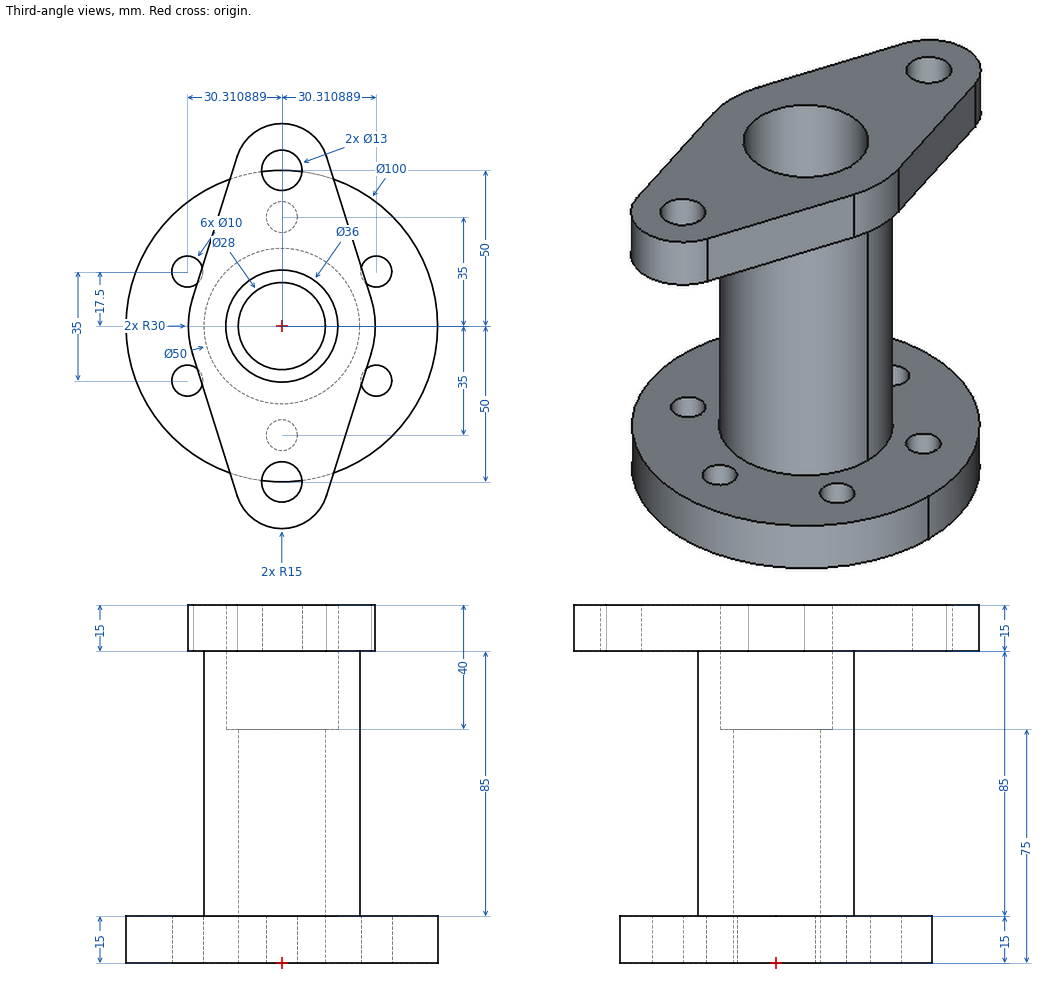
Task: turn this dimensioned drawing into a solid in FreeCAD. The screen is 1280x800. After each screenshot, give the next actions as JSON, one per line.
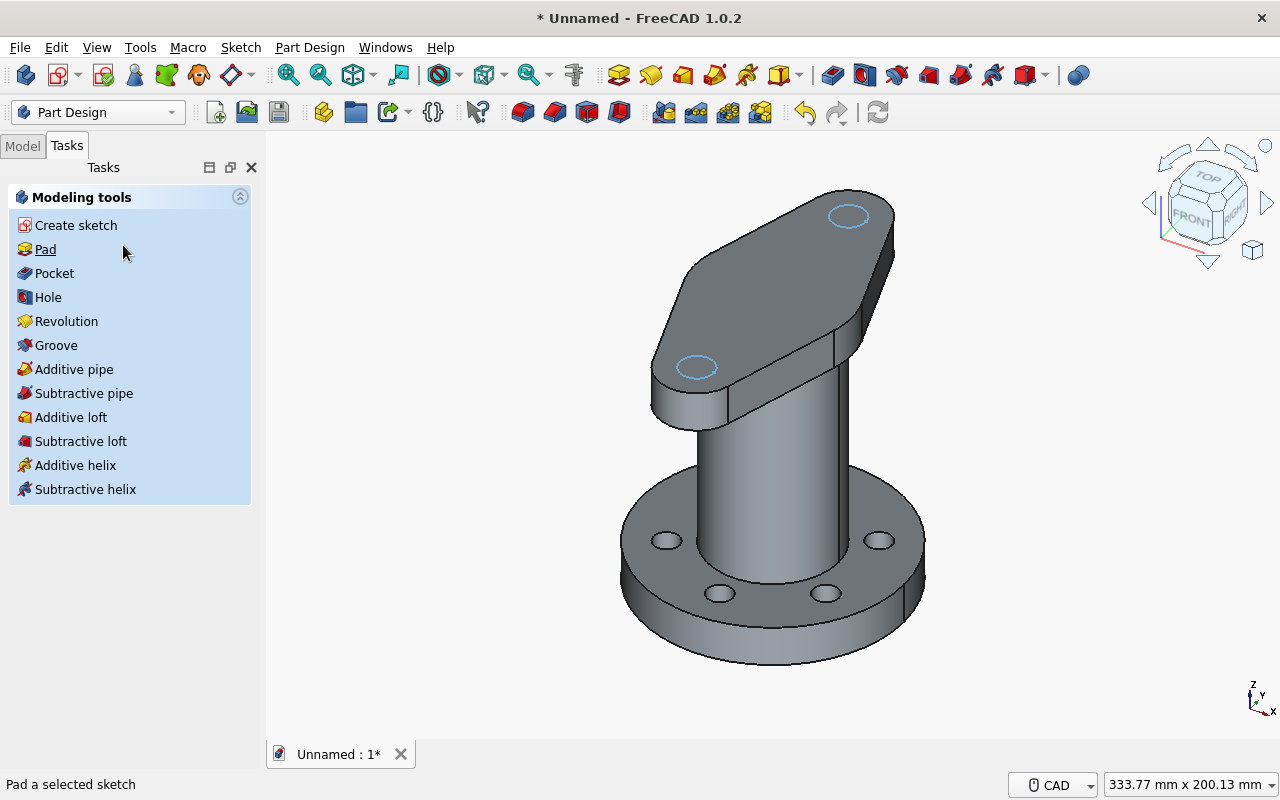
{"action": "left_click", "coordinate": [834, 76]}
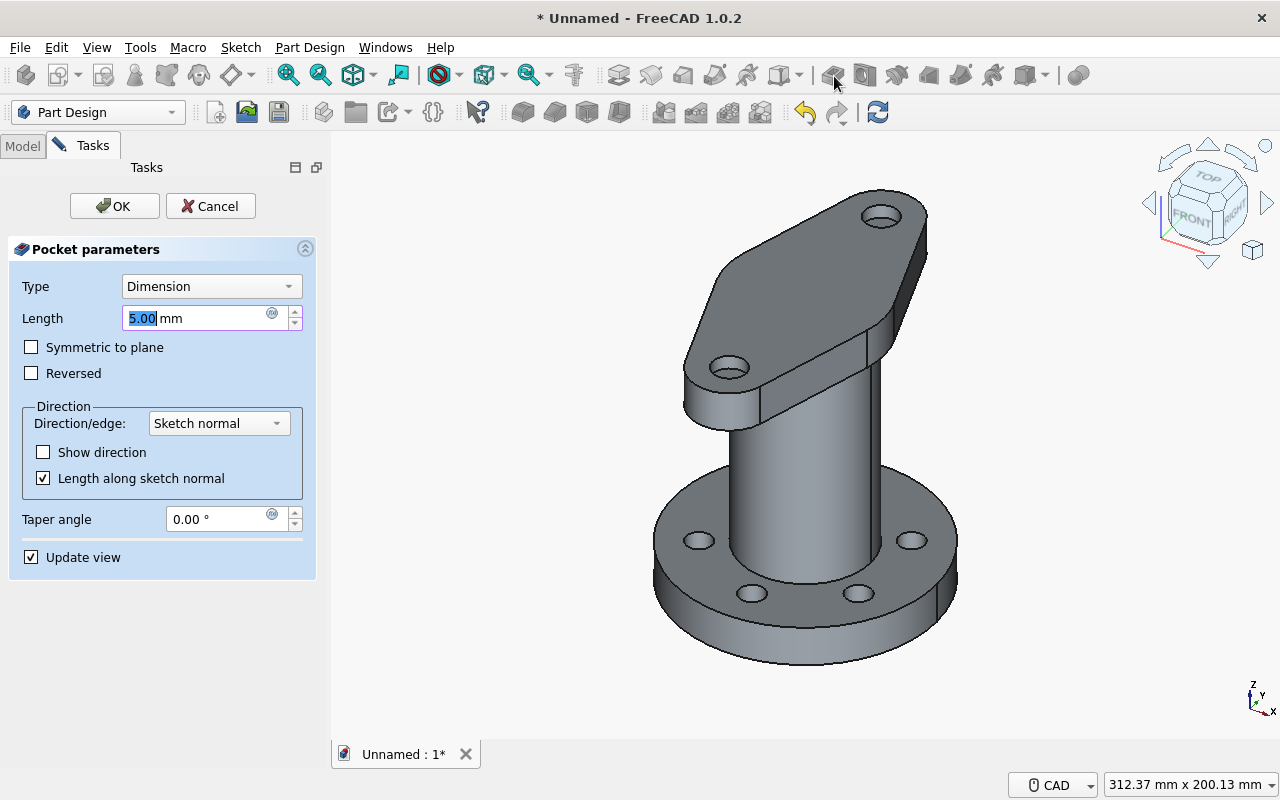
{"action": "type", "text": "15"}
{"action": "key", "text": "Tab"}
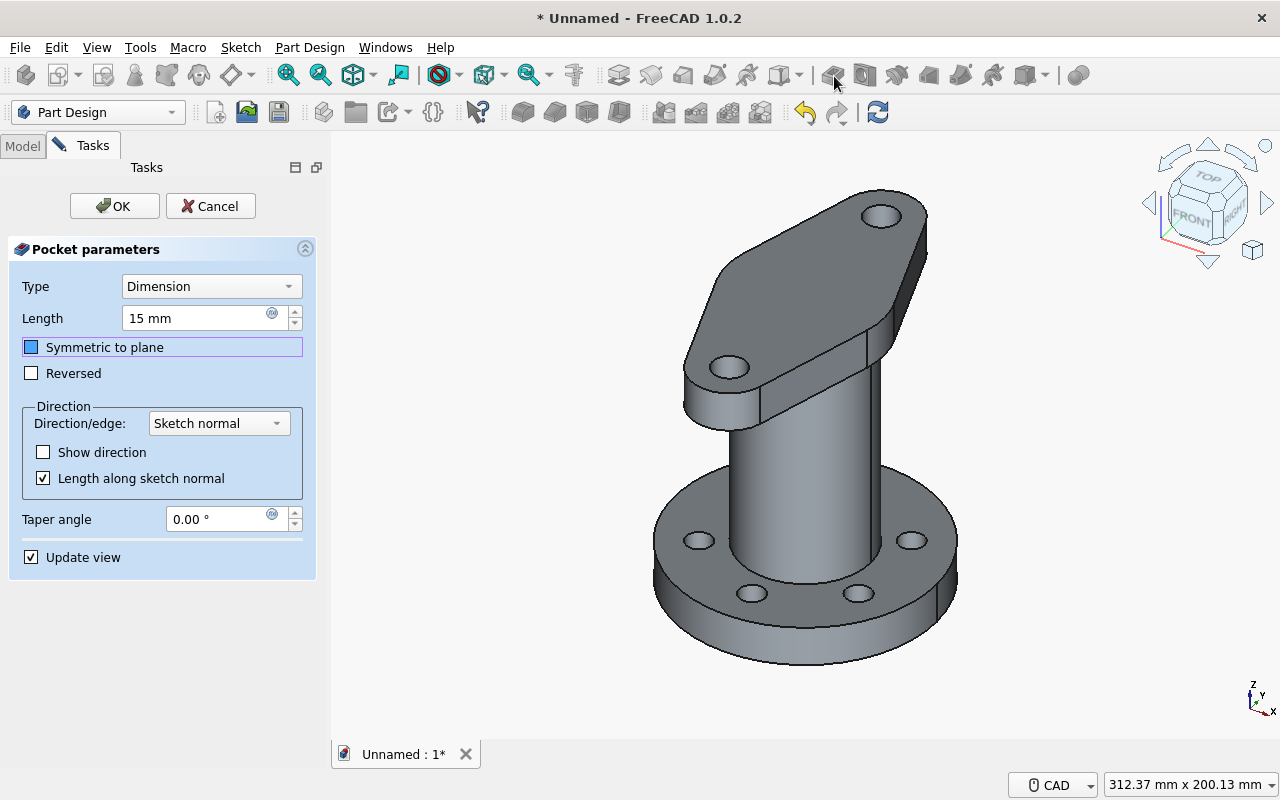
{"action": "left_click", "coordinate": [115, 206]}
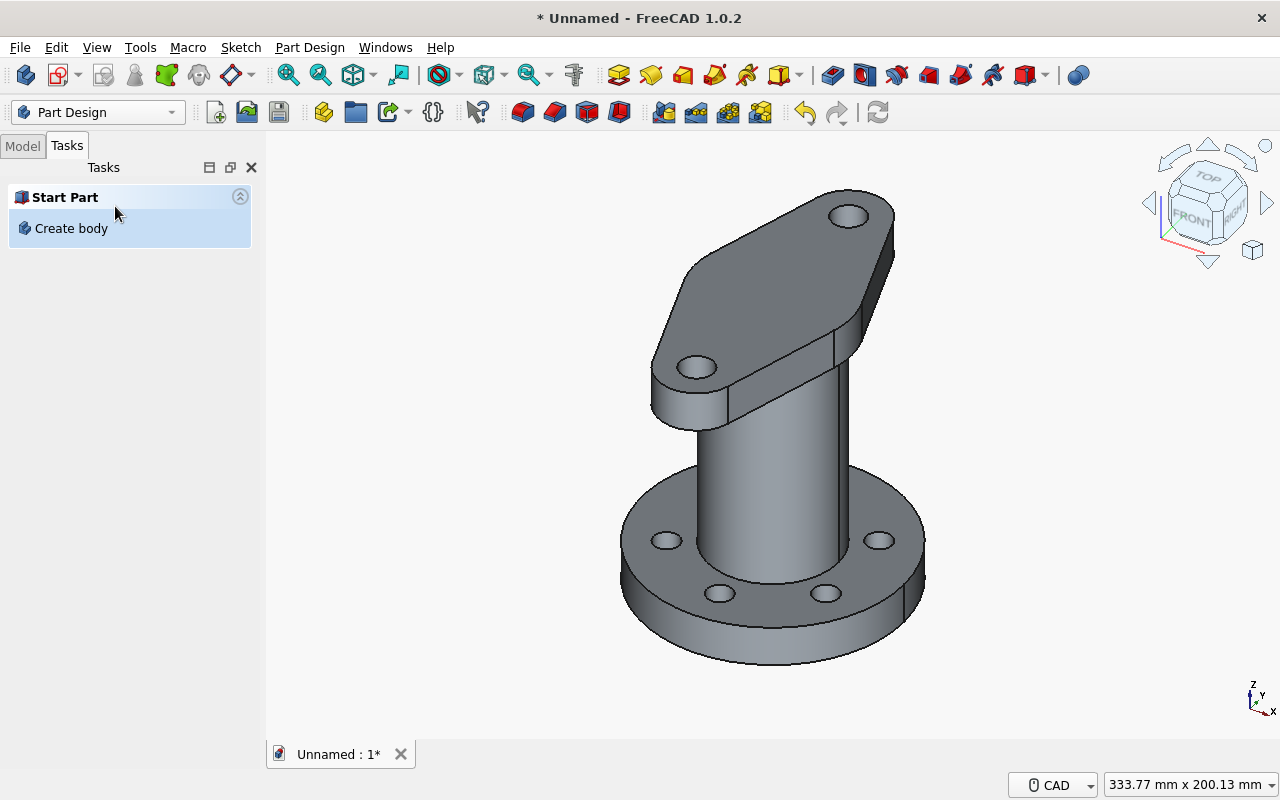
{"action": "left_click", "coordinate": [773, 291]}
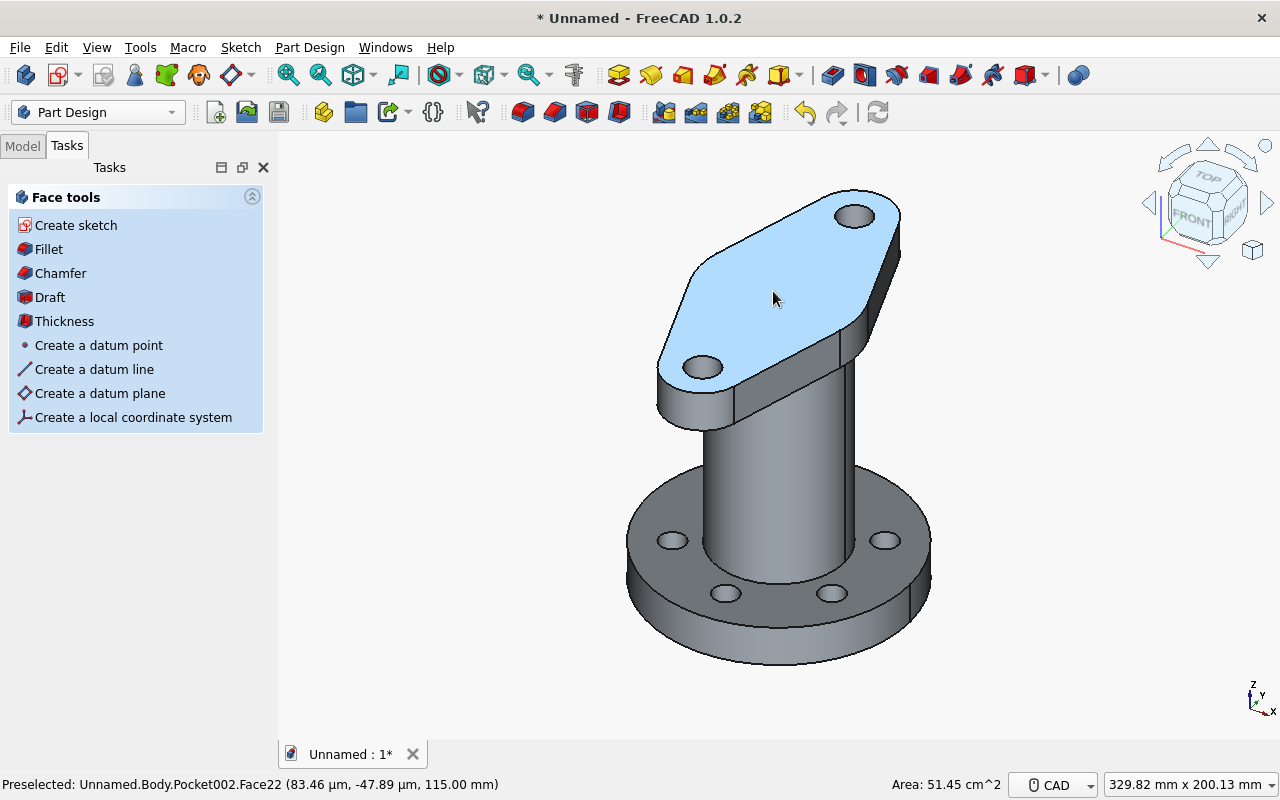
{"action": "left_click", "coordinate": [58, 76]}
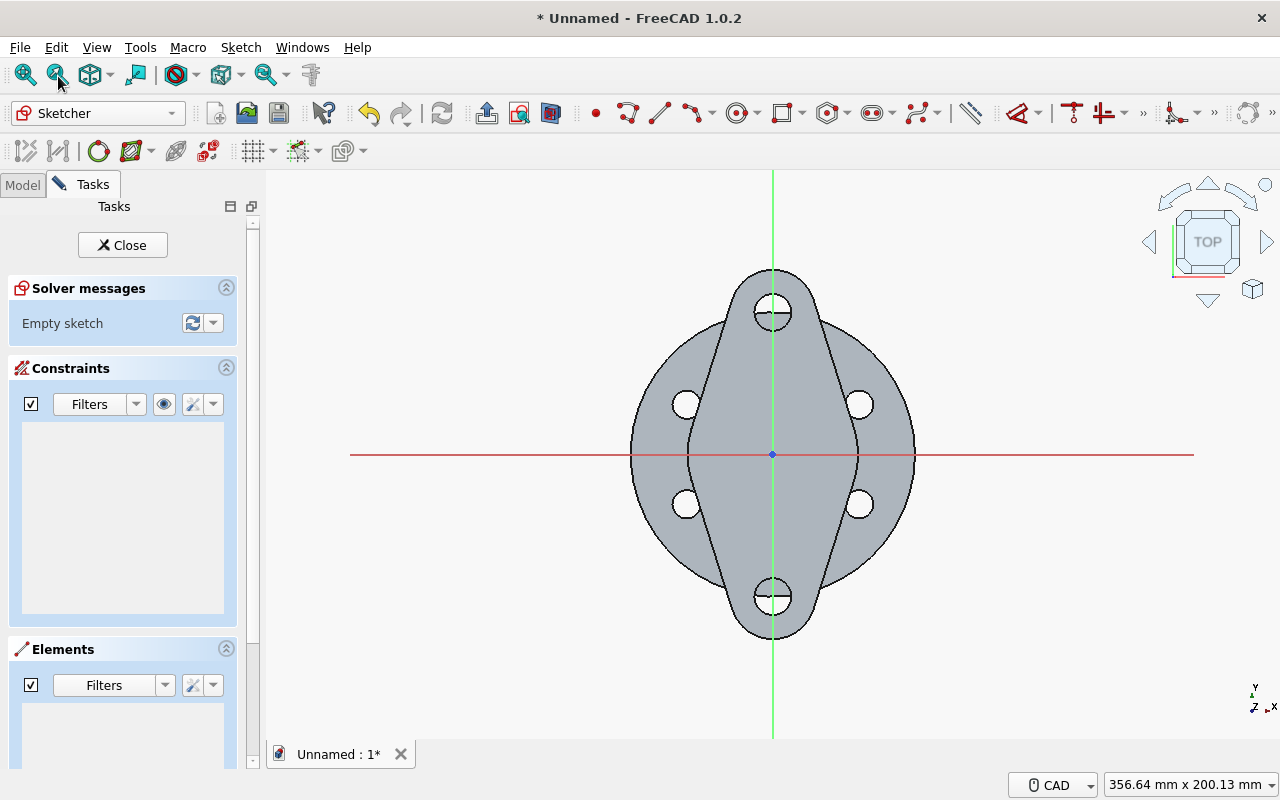
{"action": "scroll", "coordinate": [802, 455], "scroll_direction": "up", "scroll_amount": 6}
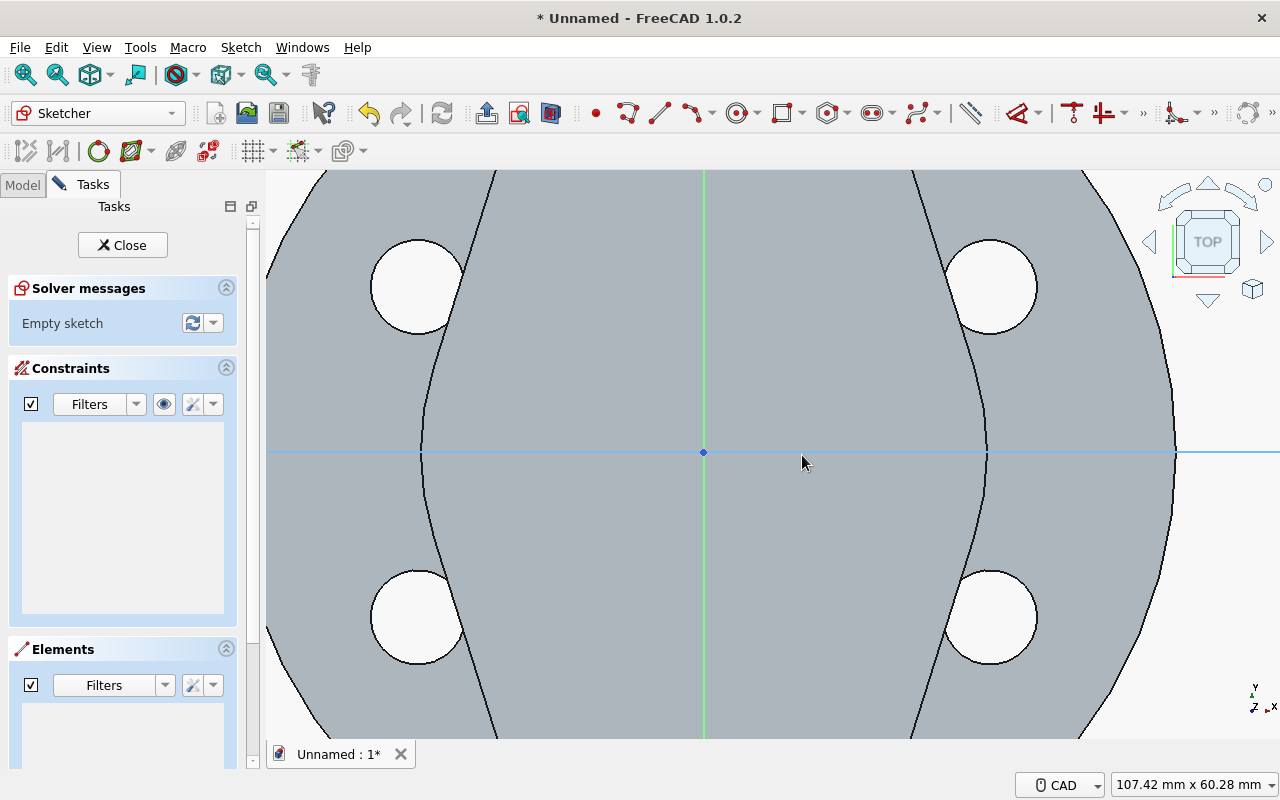
{"action": "left_click", "coordinate": [738, 114]}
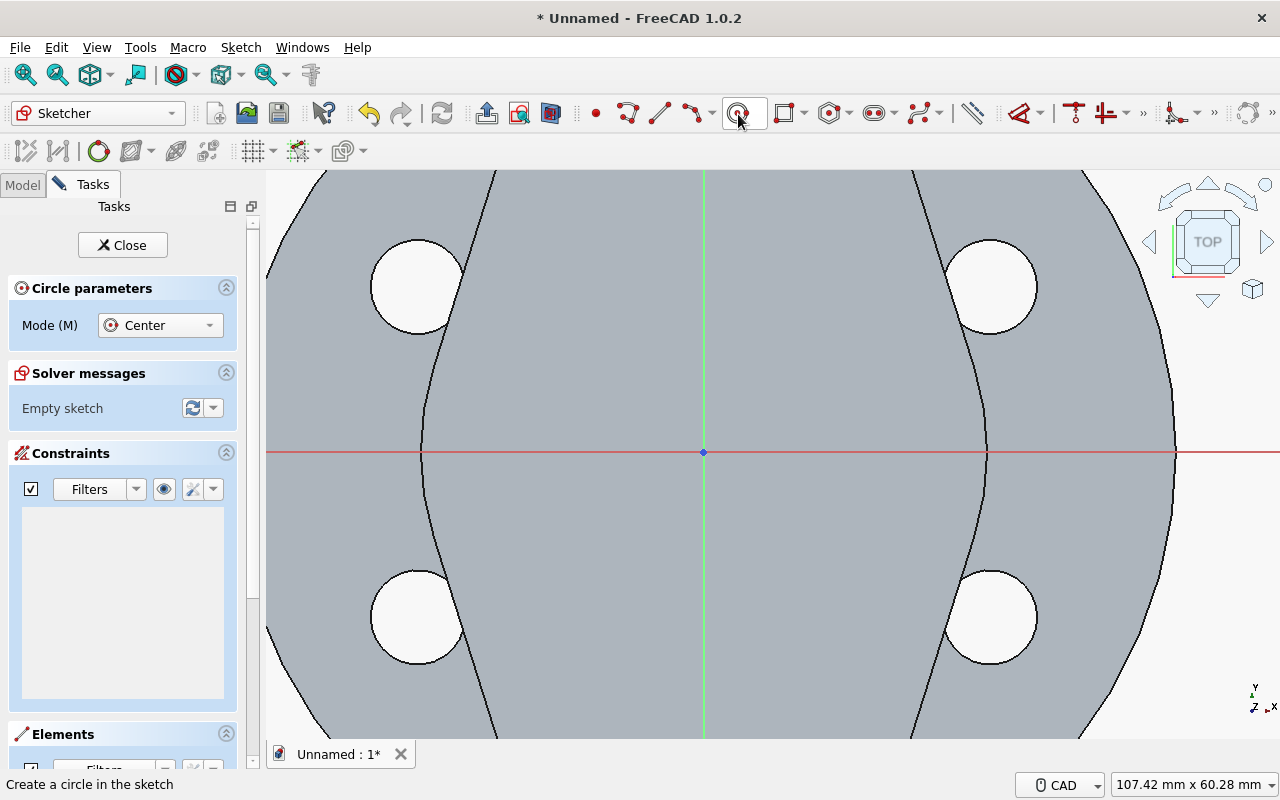
{"action": "left_click", "coordinate": [704, 452]}
{"action": "mouse_move", "coordinate": [824, 332]}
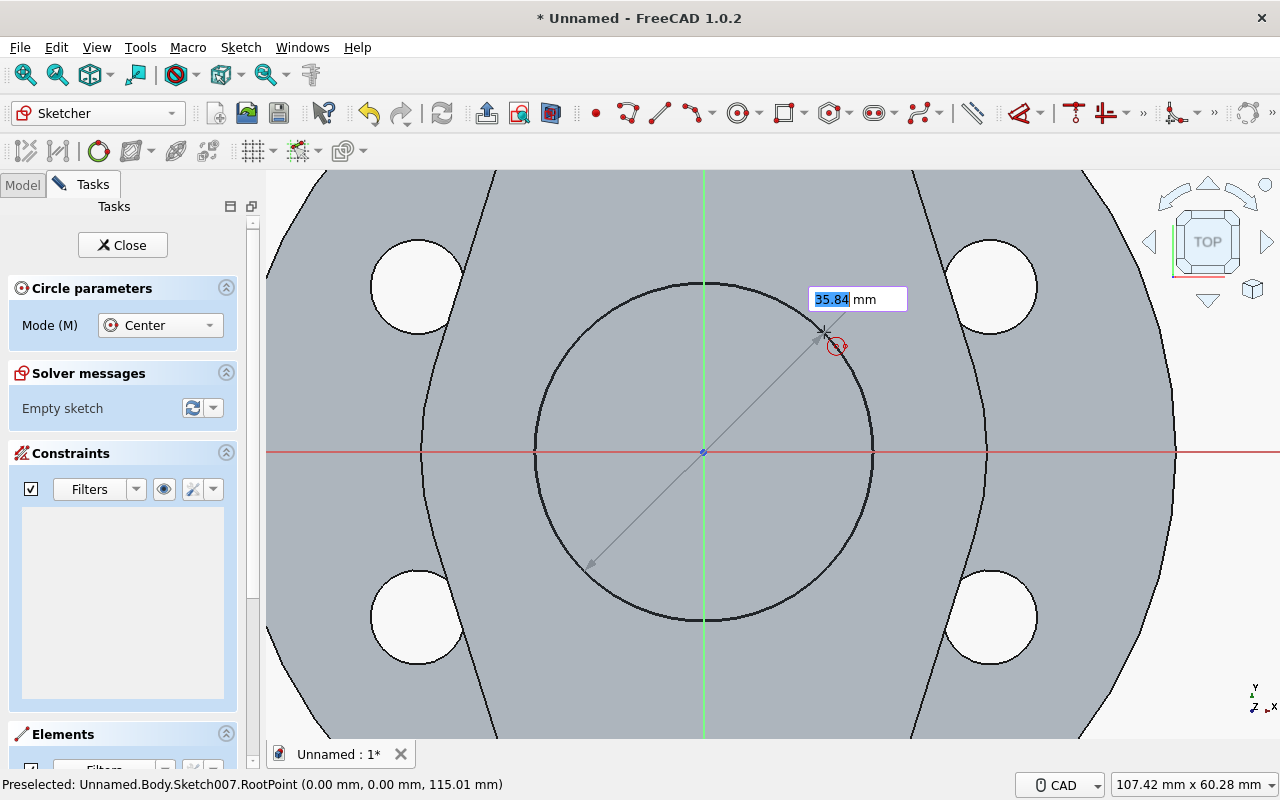
{"action": "type", "text": "36"}
{"action": "key", "text": "Return"}
{"action": "key", "text": "Escape"}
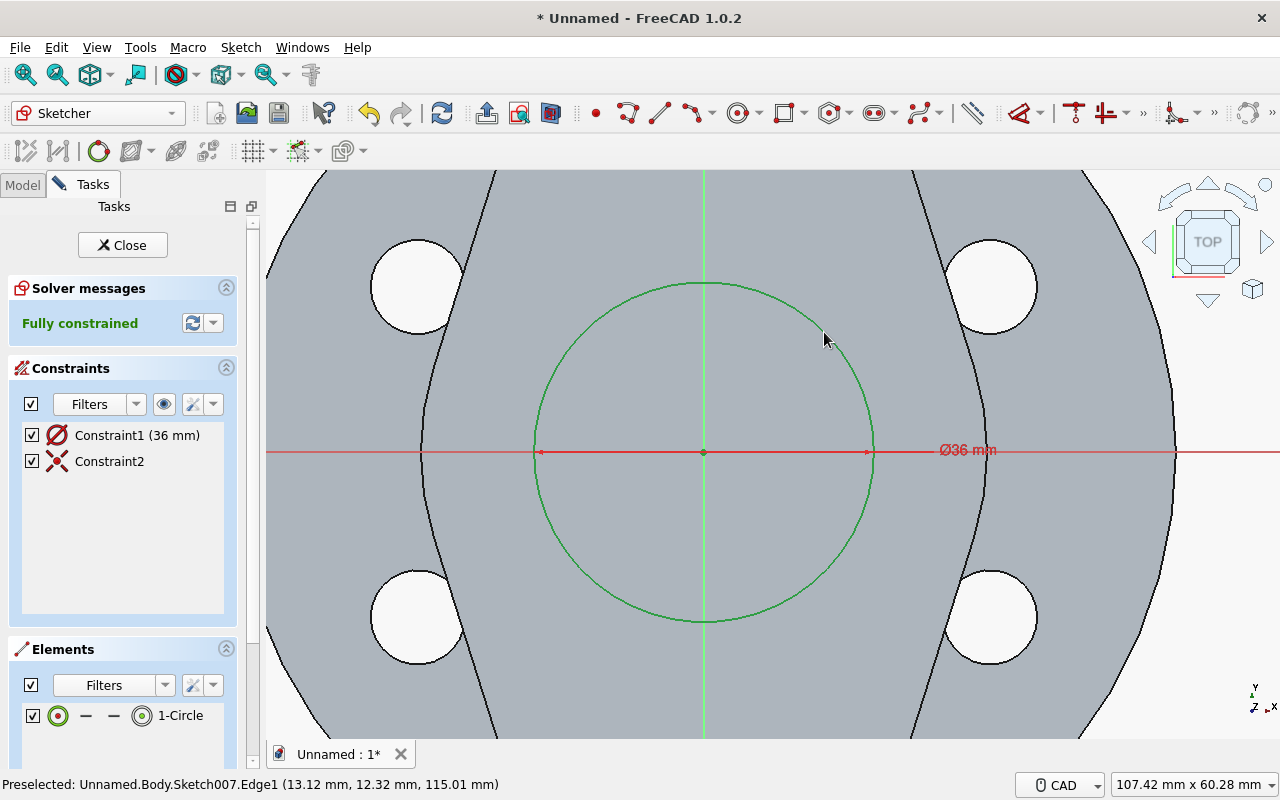
{"action": "left_click", "coordinate": [123, 245]}